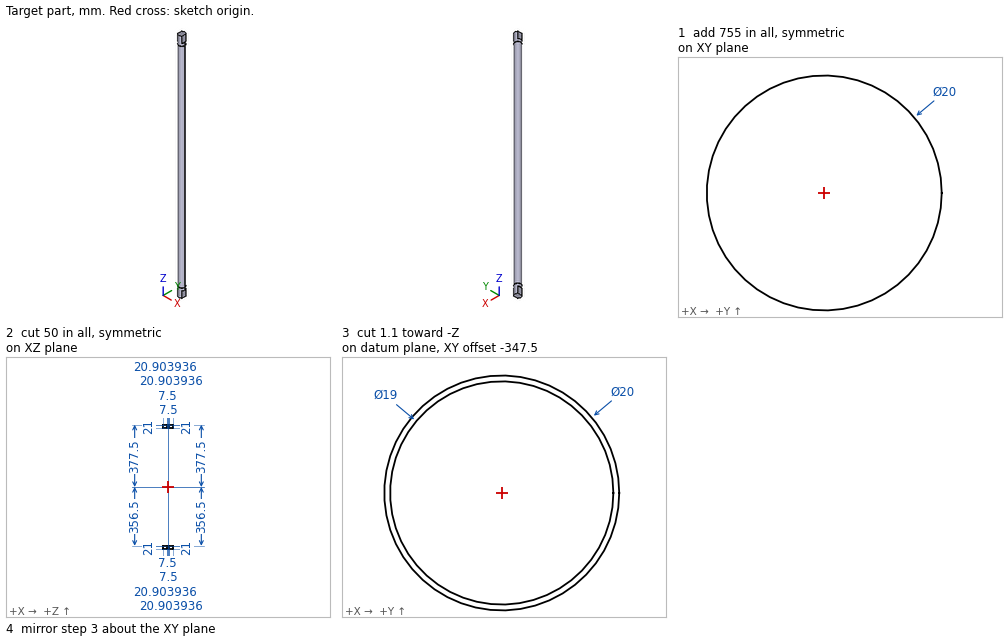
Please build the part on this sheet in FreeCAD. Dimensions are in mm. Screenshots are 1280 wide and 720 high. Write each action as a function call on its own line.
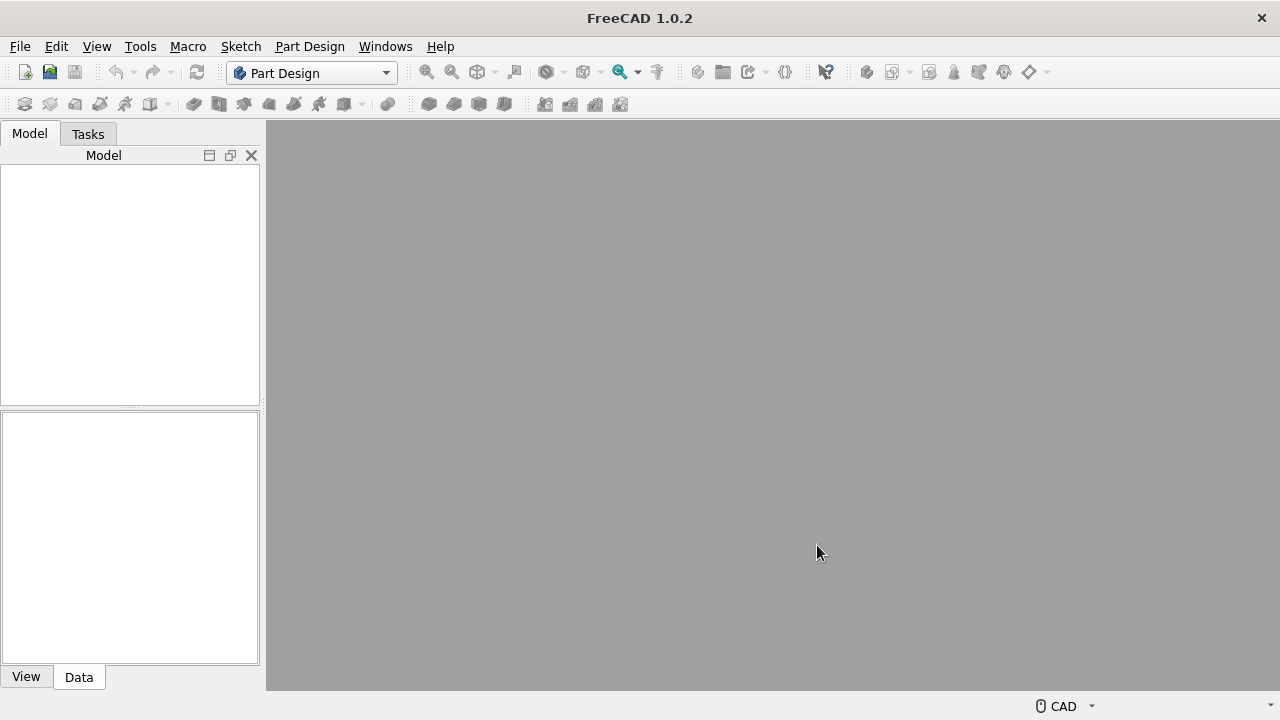
key(ctrl+n)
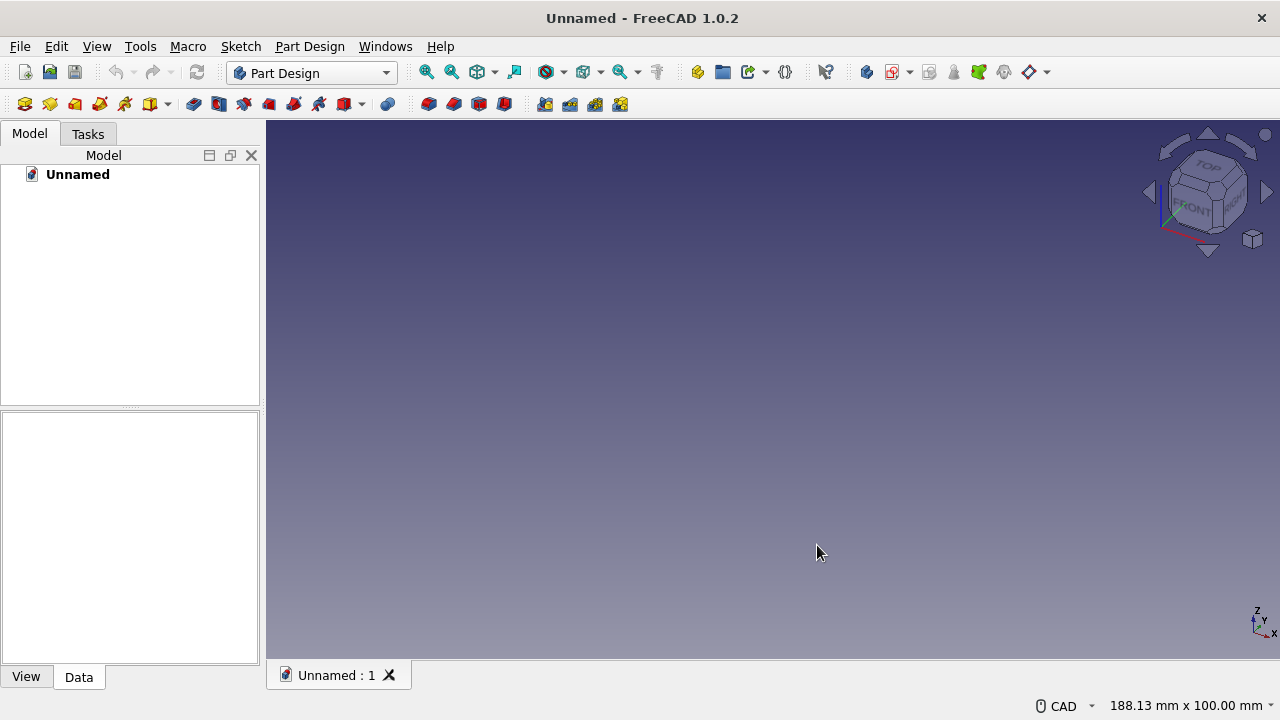
click(892, 72)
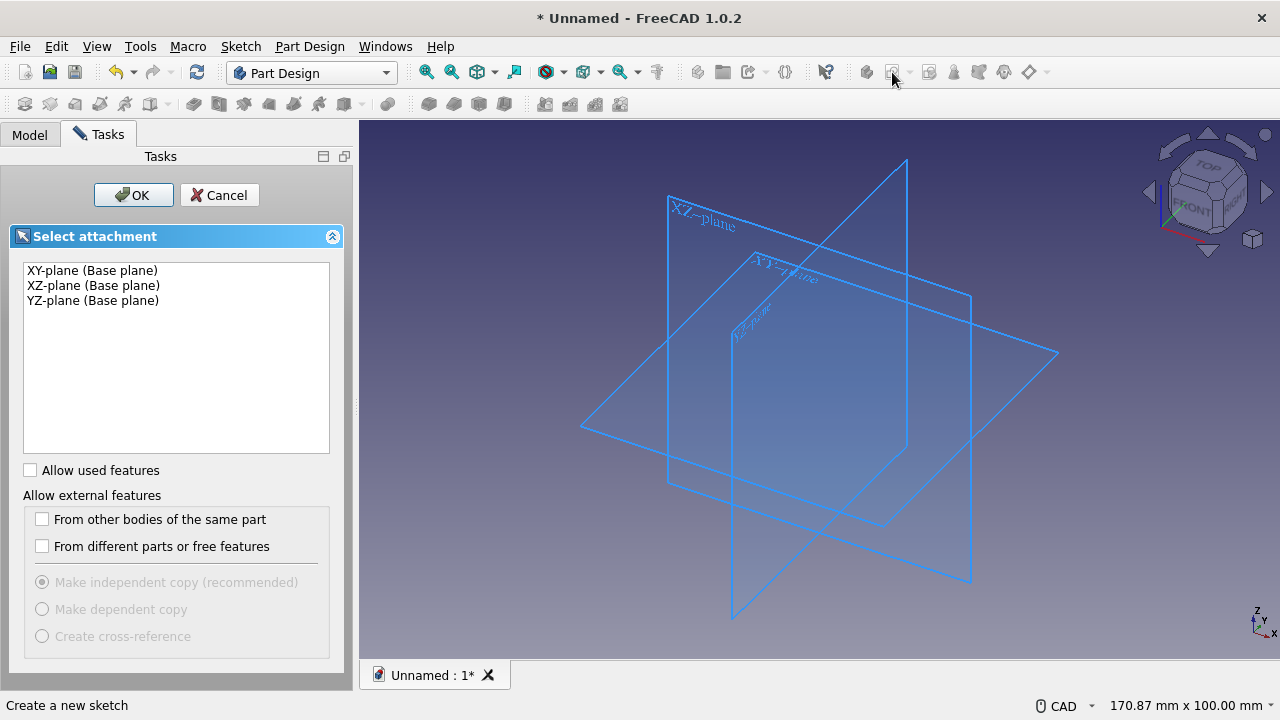
click(84, 270)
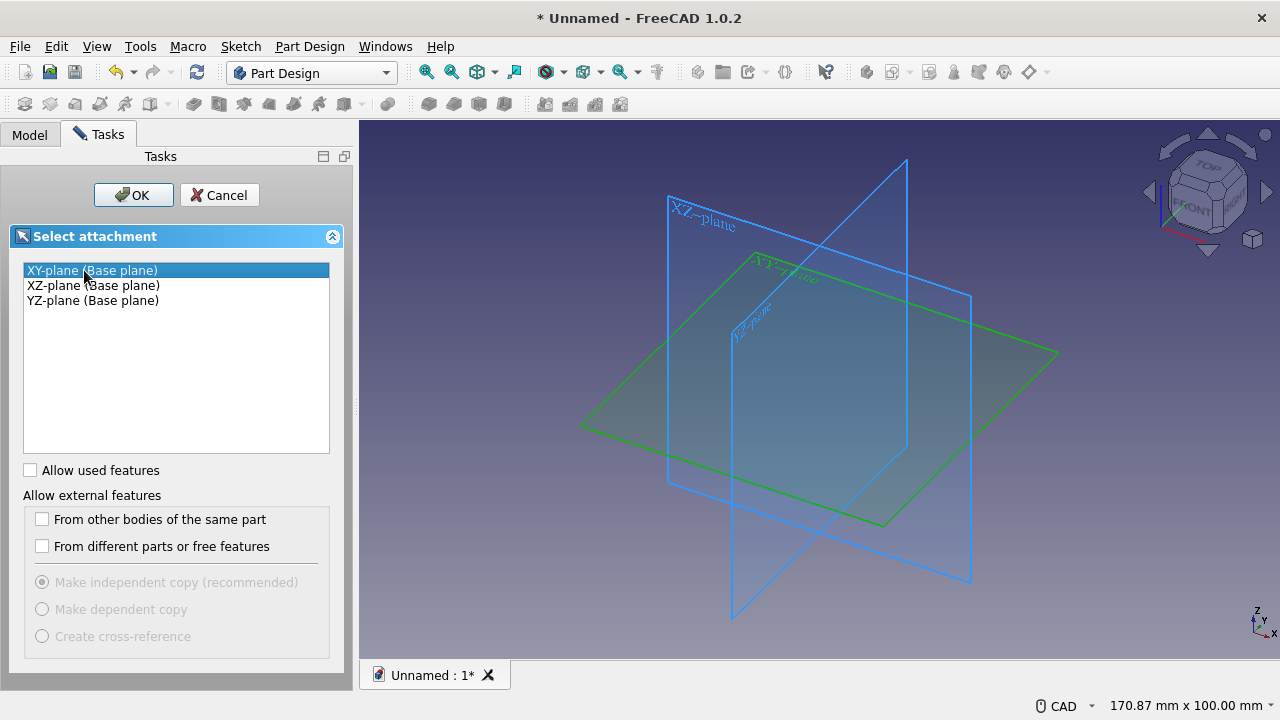
click(134, 195)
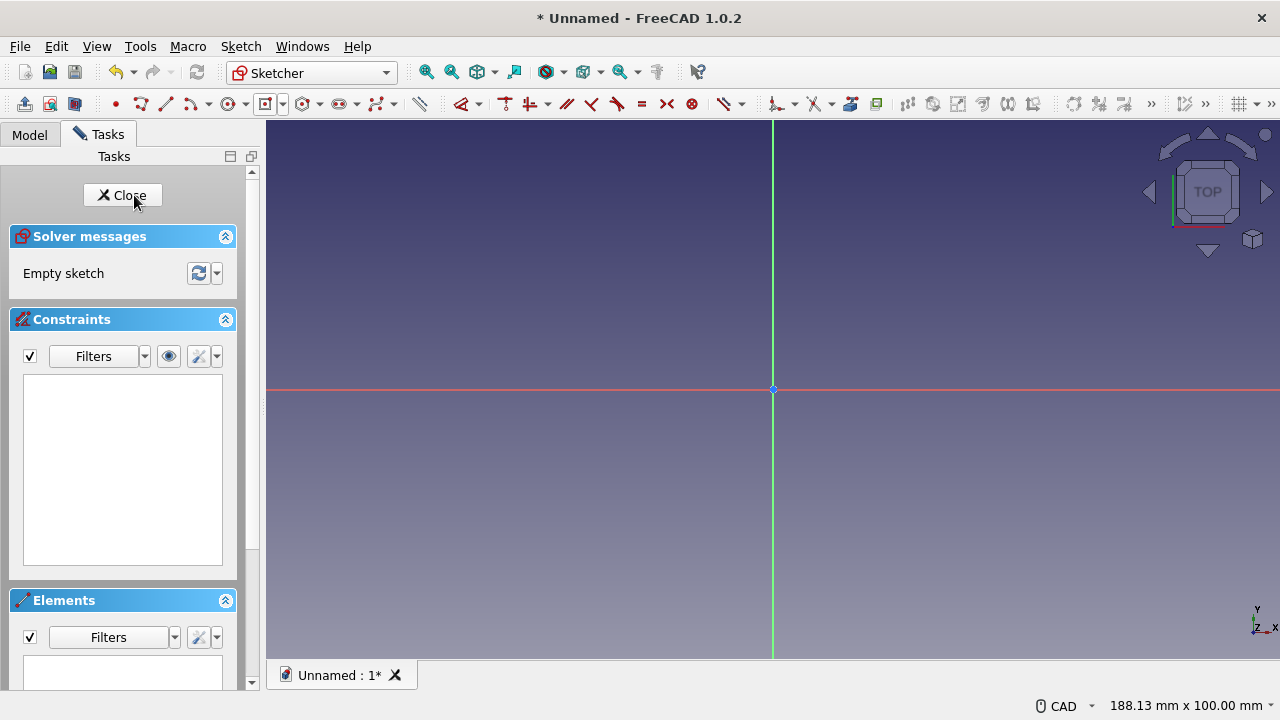
scroll(803, 390, up, 6)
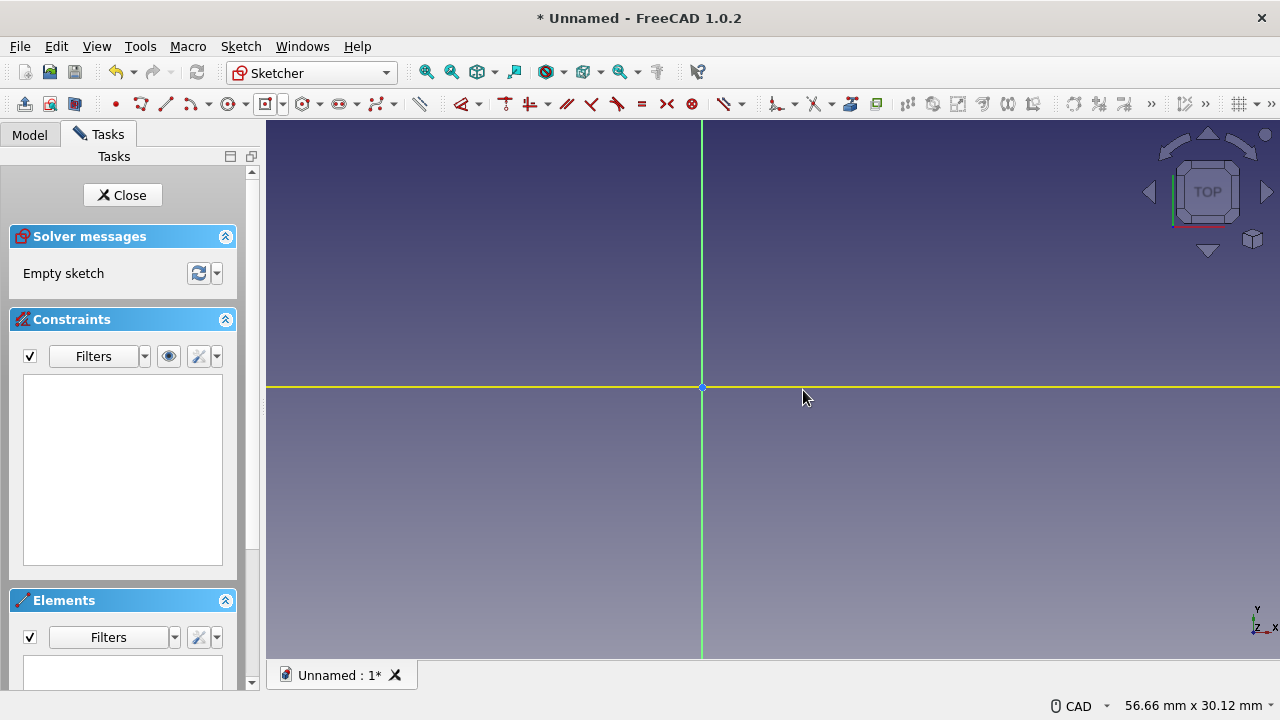
key(g)
key(c)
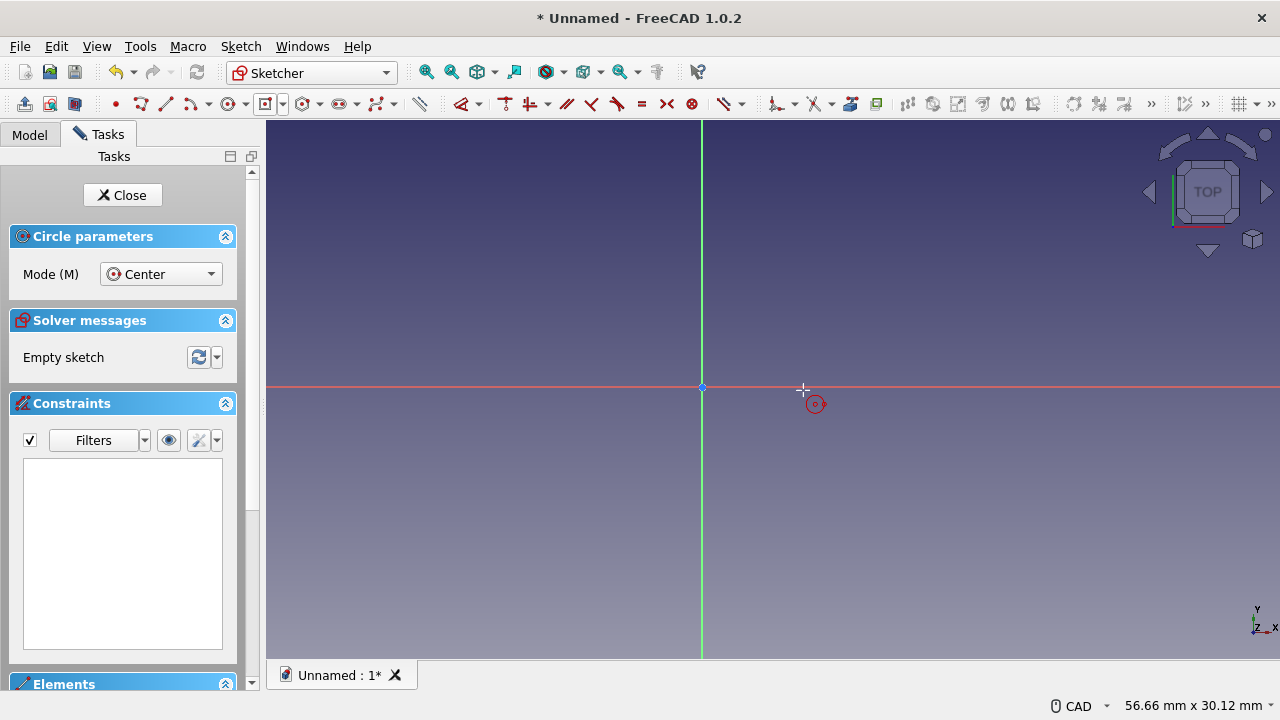
click(702, 387)
move(829, 261)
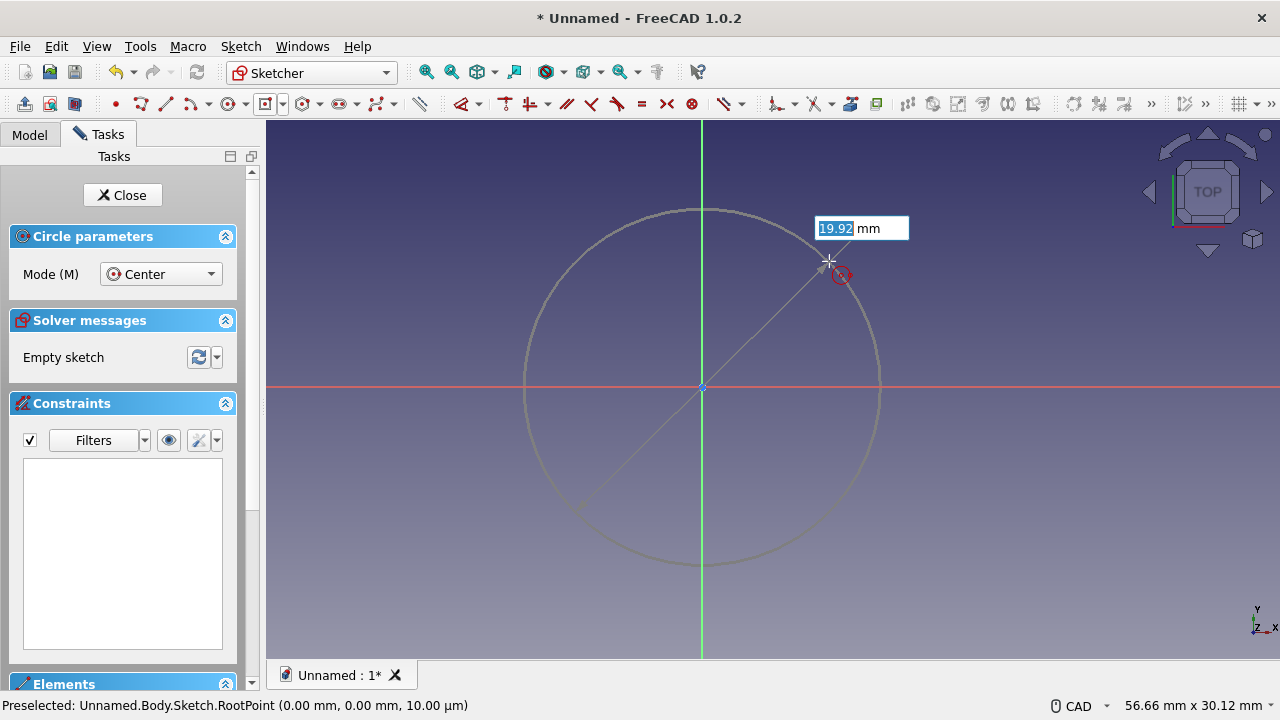
text(20)
key(Return)
key(Escape)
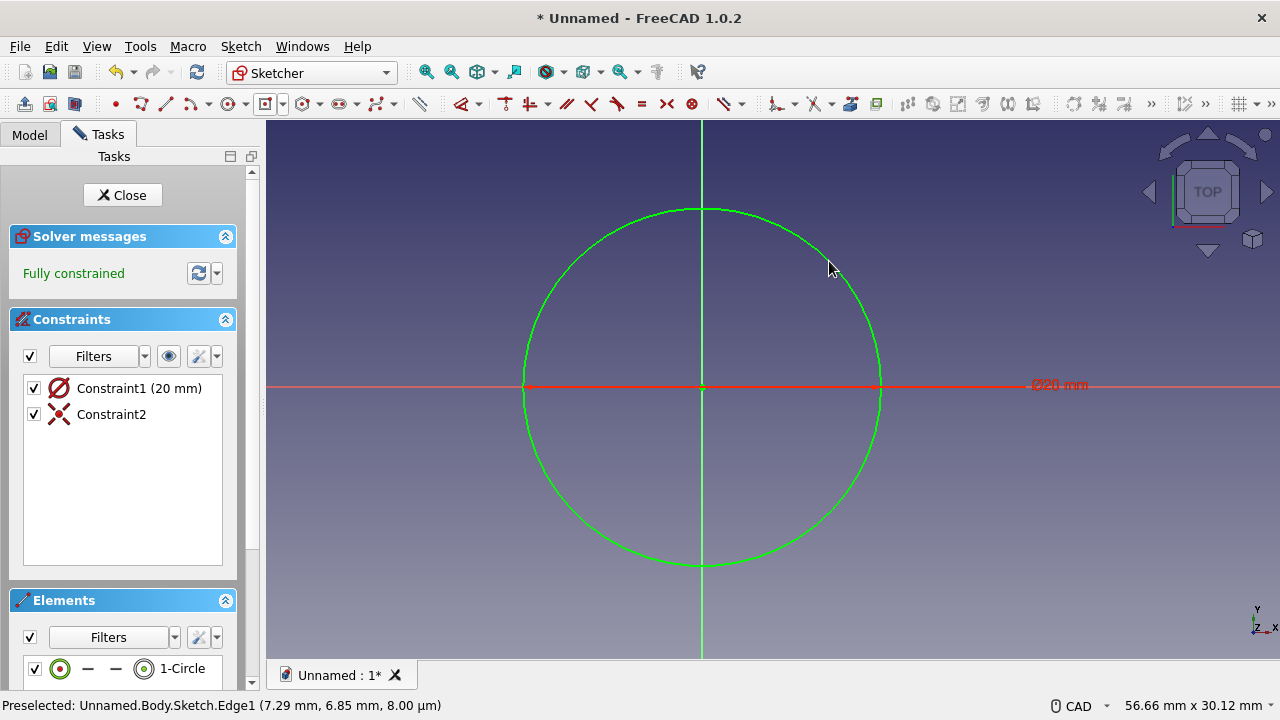
click(123, 195)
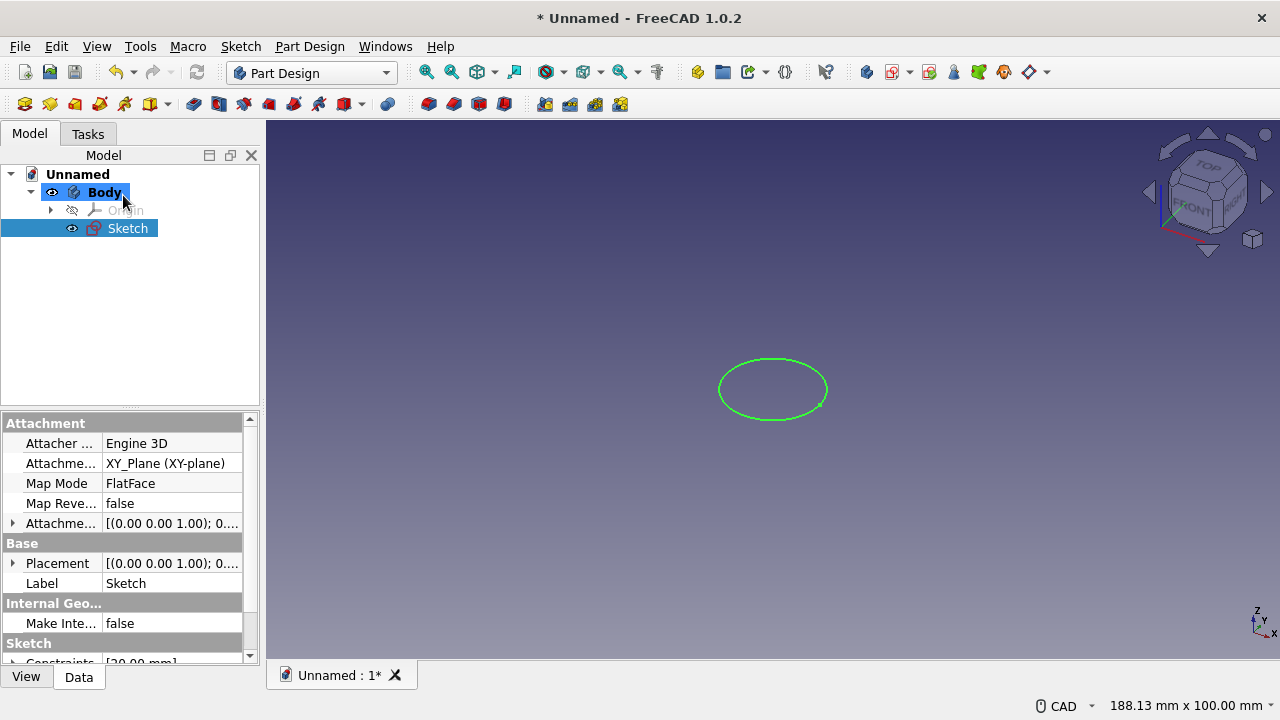
click(25, 104)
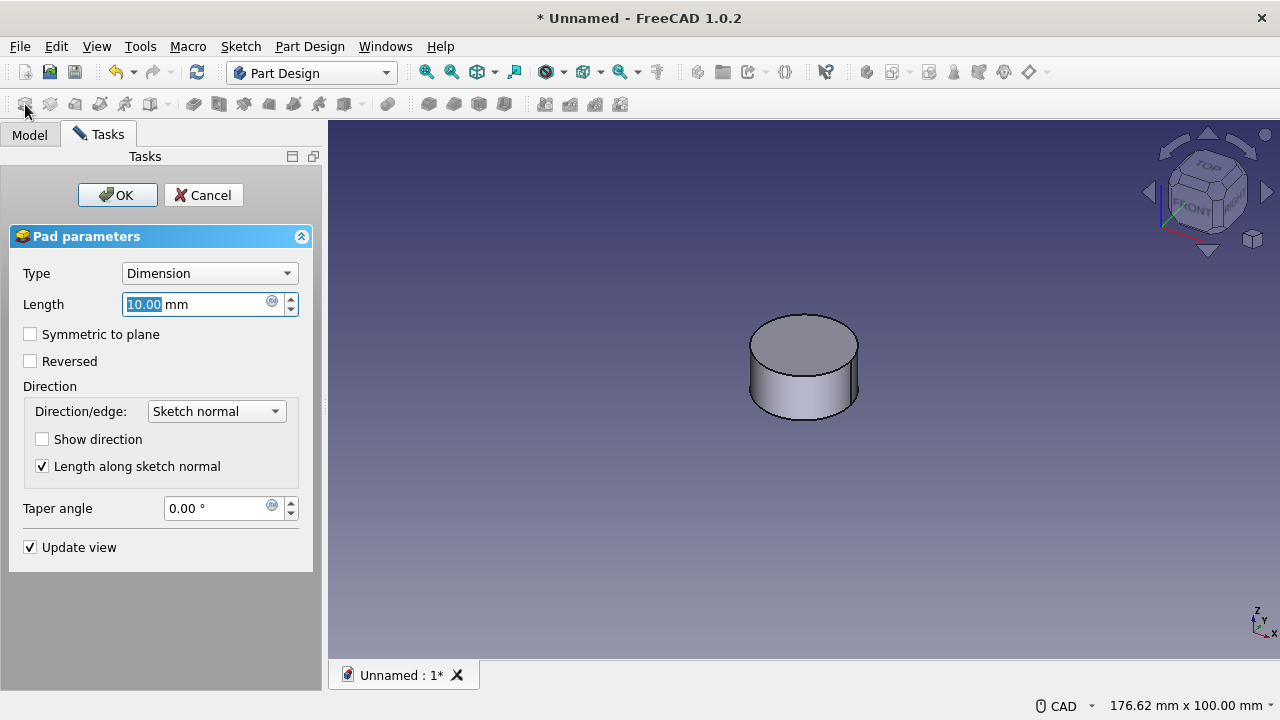
text(755)
key(Tab)